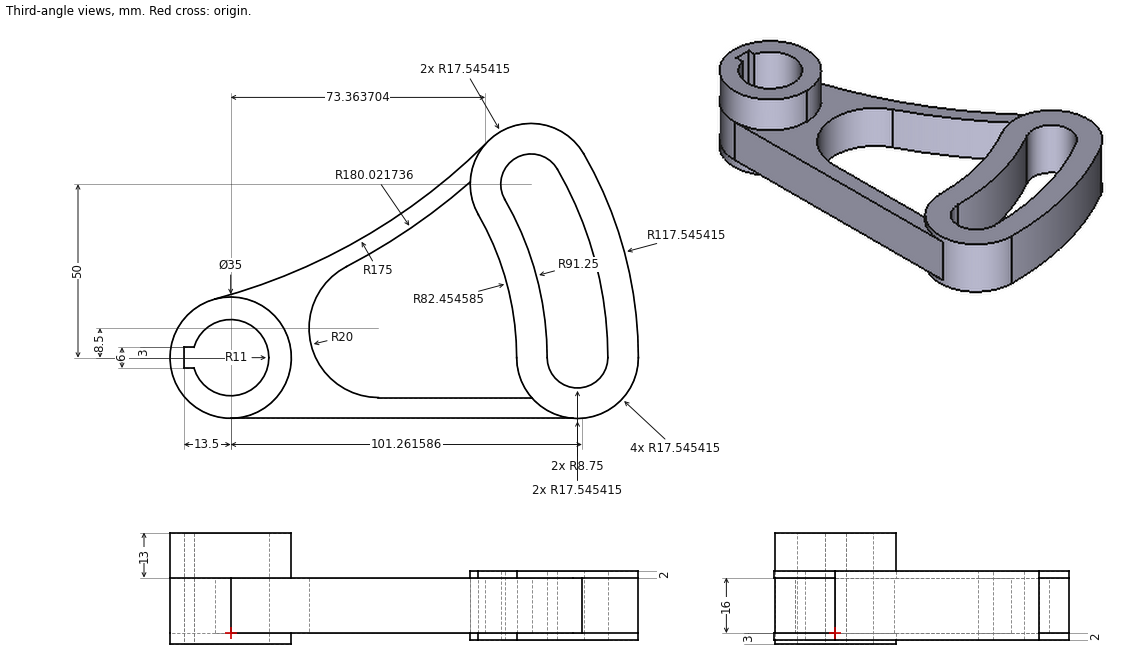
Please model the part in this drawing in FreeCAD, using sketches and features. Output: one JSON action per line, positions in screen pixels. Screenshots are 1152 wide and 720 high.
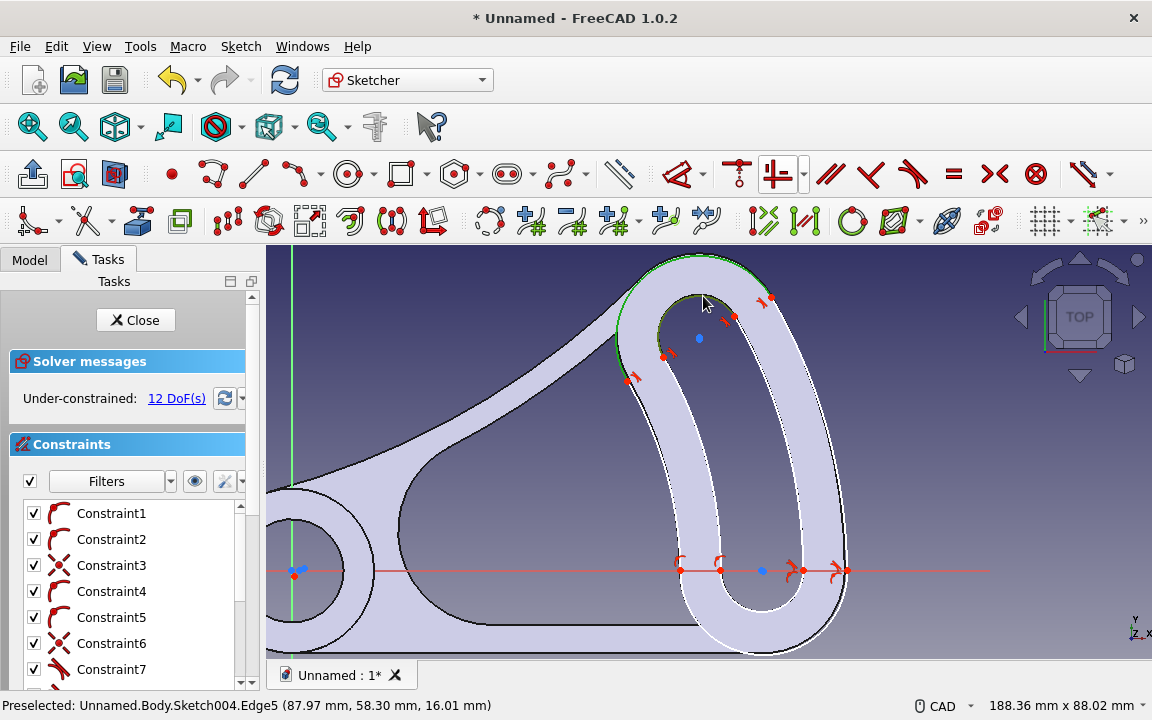
{"action": "left_click", "coordinate": [737, 174]}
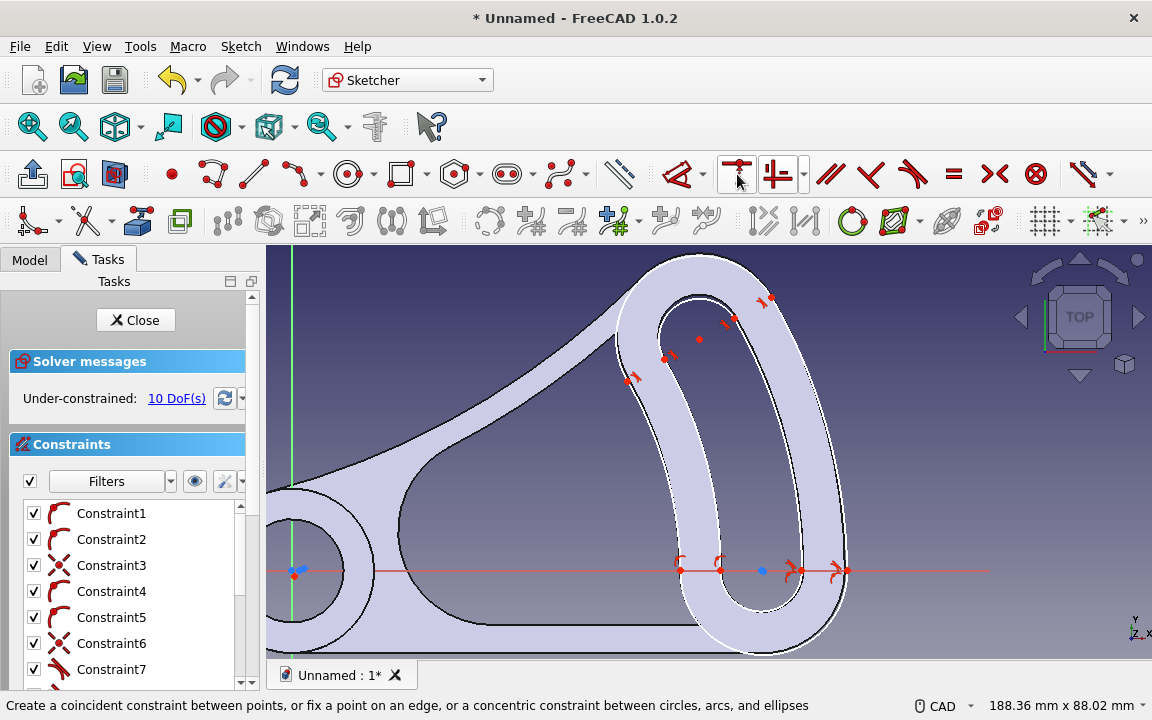
{"action": "left_click", "coordinate": [840, 485]}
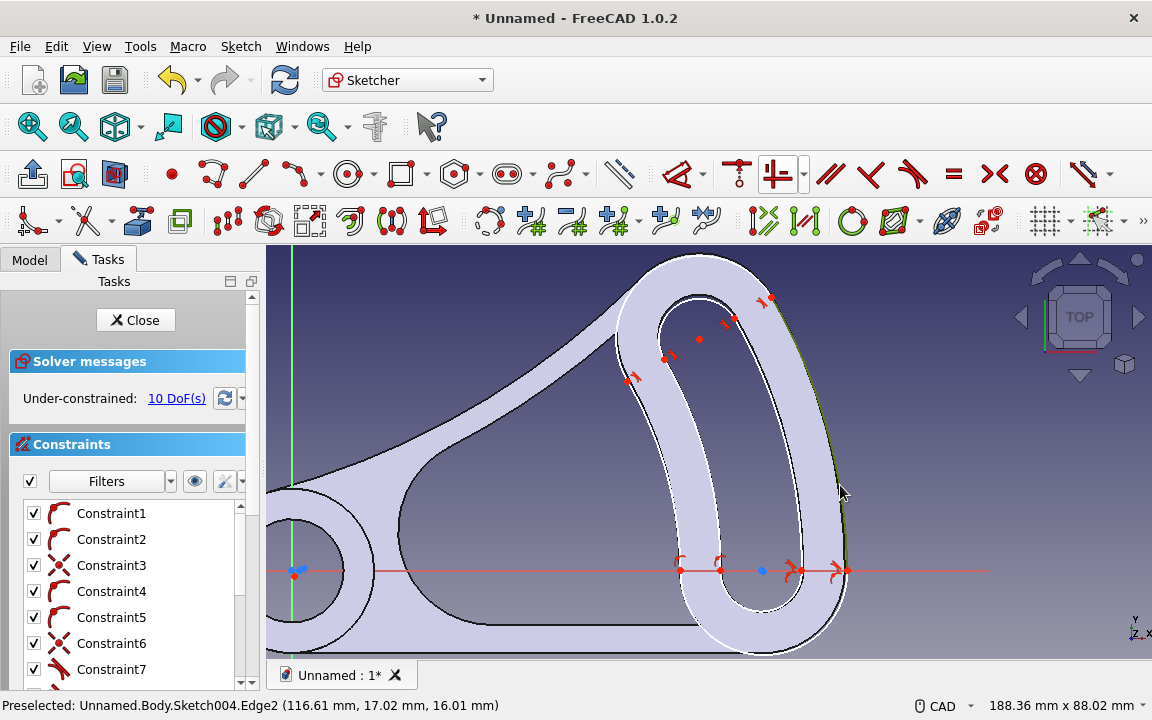
{"action": "left_click", "coordinate": [796, 492]}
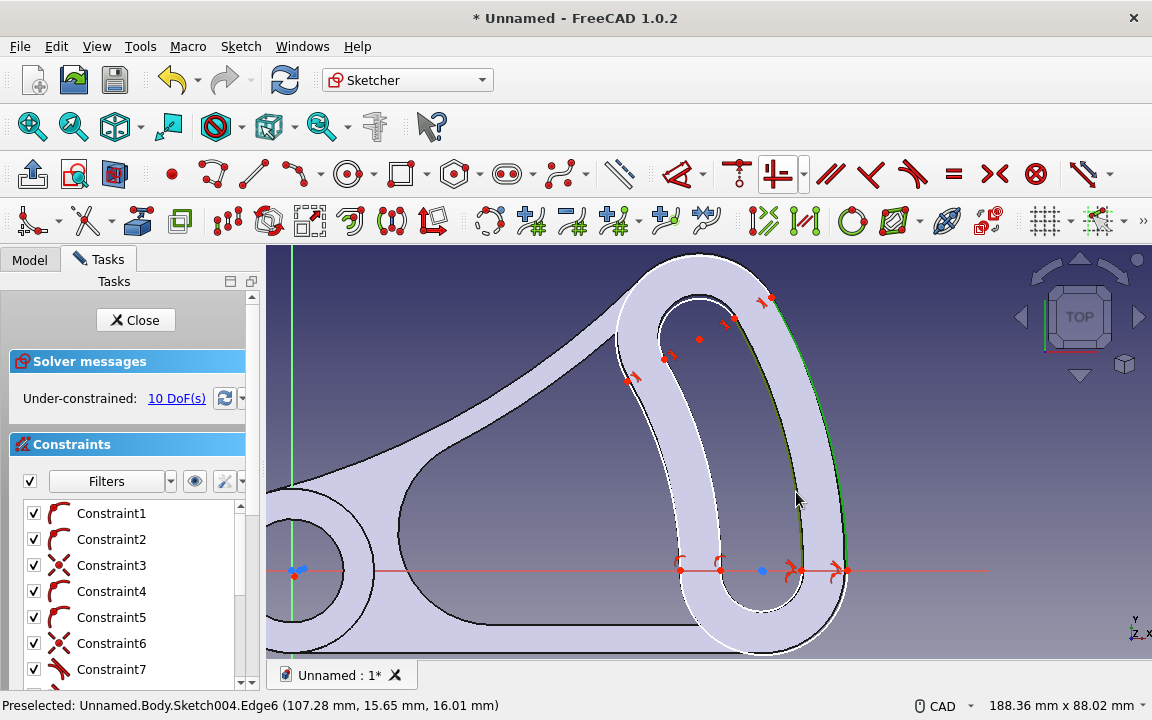
{"action": "left_click", "coordinate": [737, 174]}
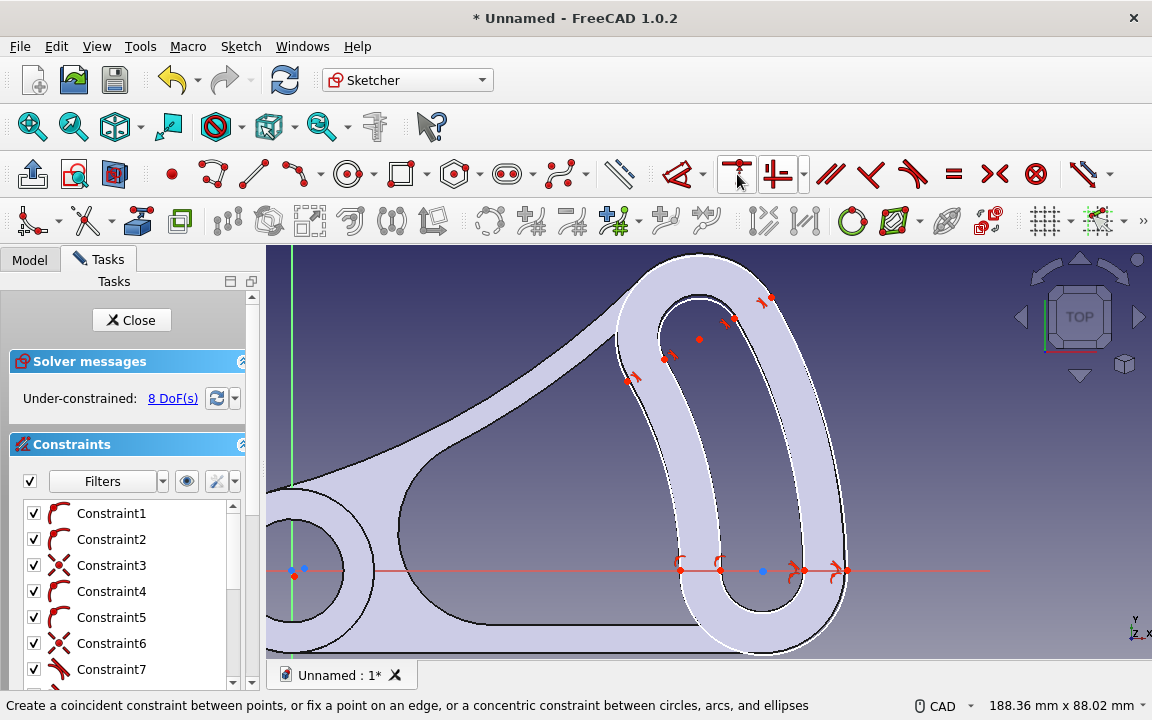
{"action": "left_click", "coordinate": [840, 485]}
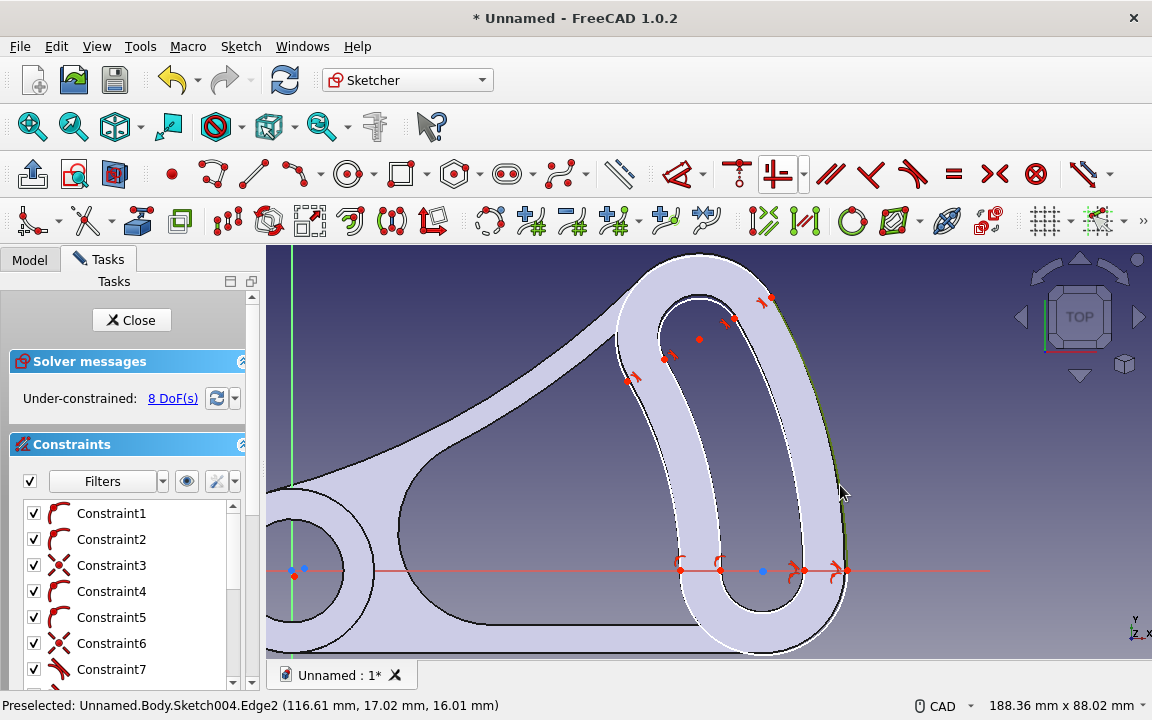
{"action": "left_click", "coordinate": [716, 505]}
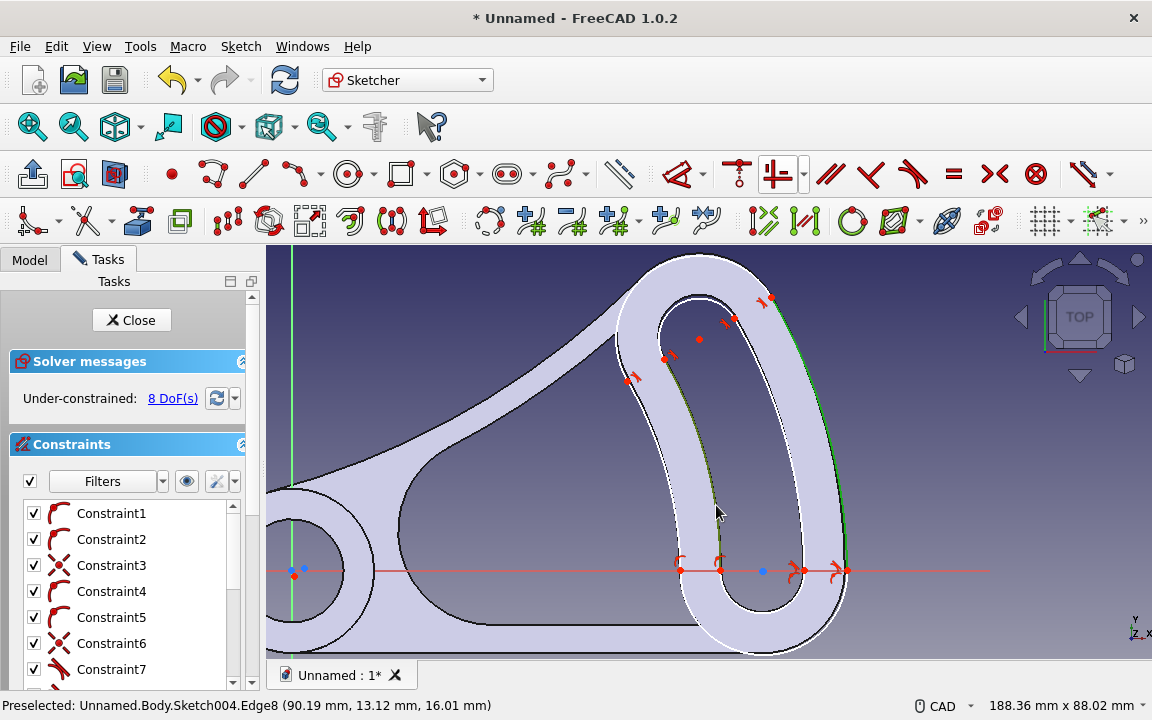
{"action": "left_click", "coordinate": [737, 174]}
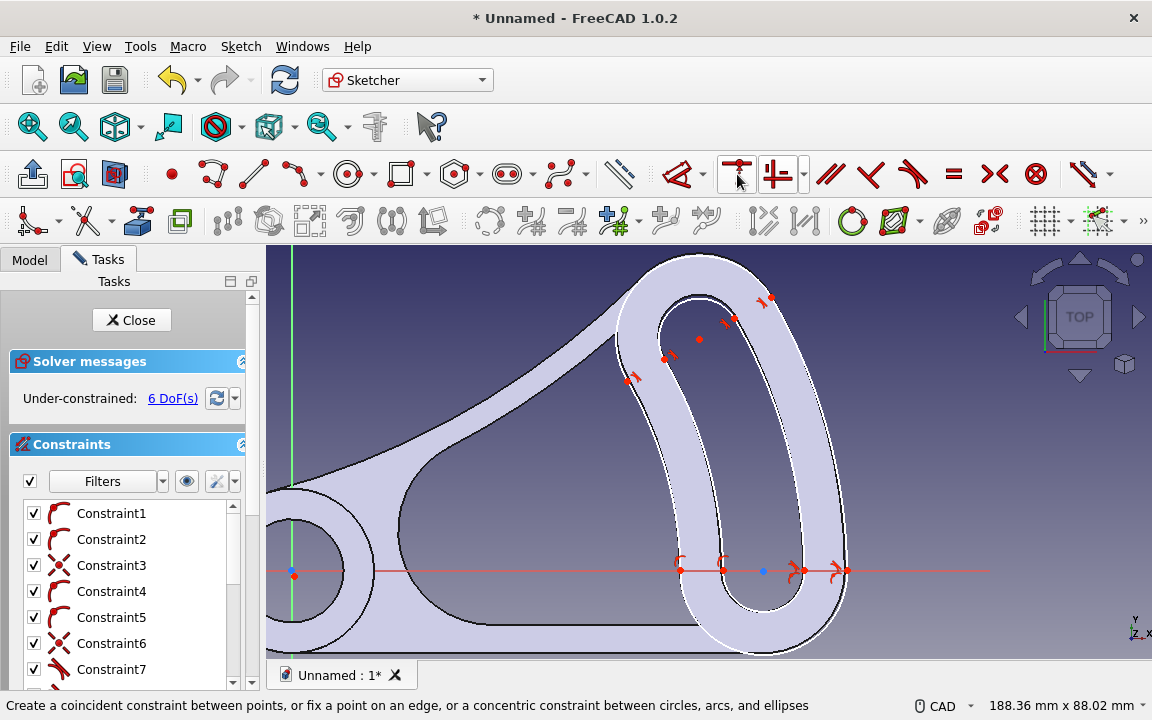
{"action": "scroll", "coordinate": [787, 438], "scroll_direction": "down", "scroll_amount": 2}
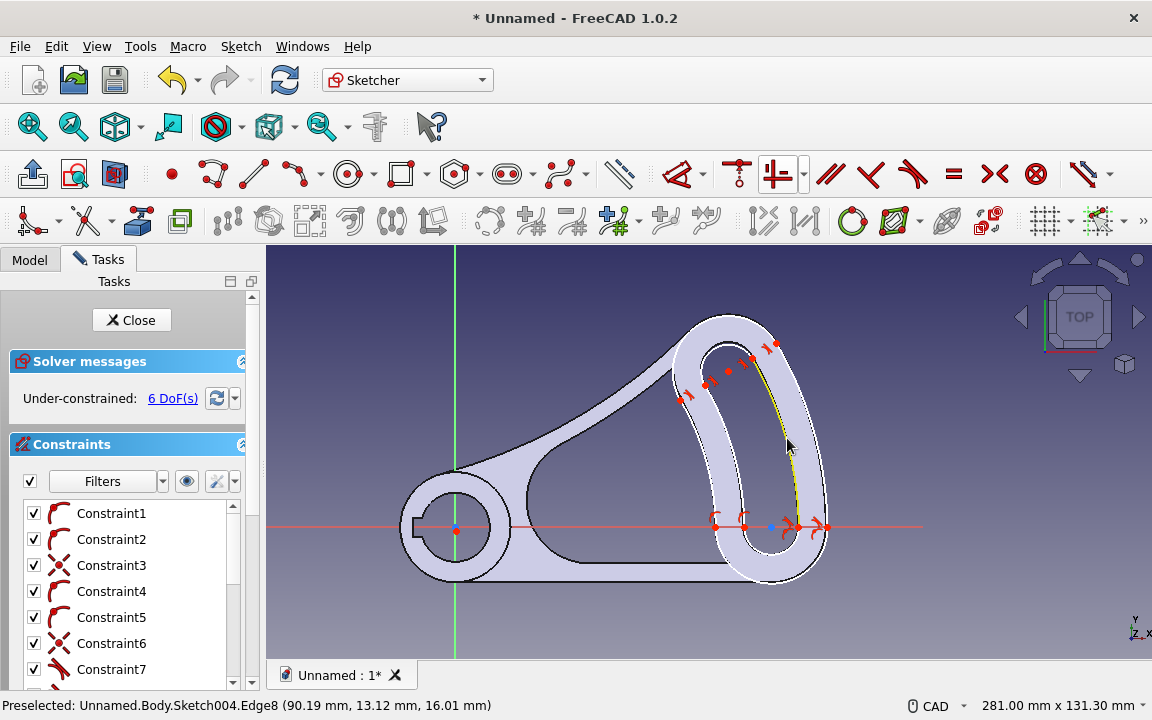
{"action": "scroll", "coordinate": [456, 529], "scroll_direction": "up", "scroll_amount": 2}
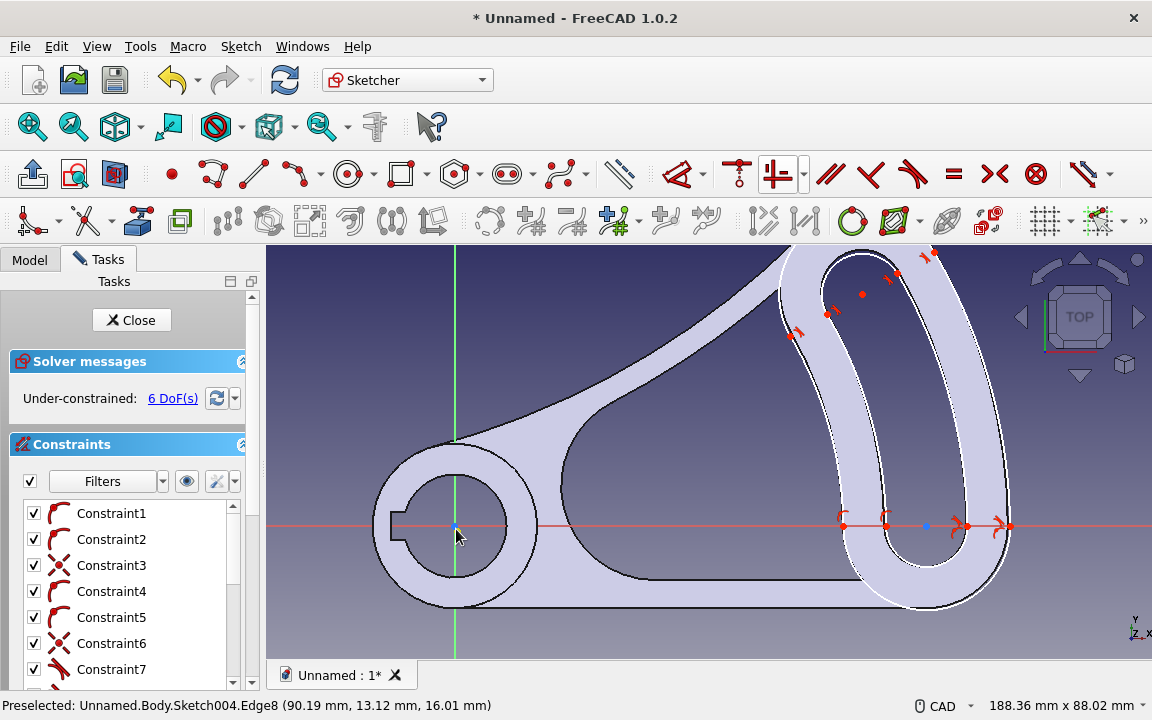
{"action": "left_click_drag", "start_coordinate": [445, 516], "coordinate": [467, 542]}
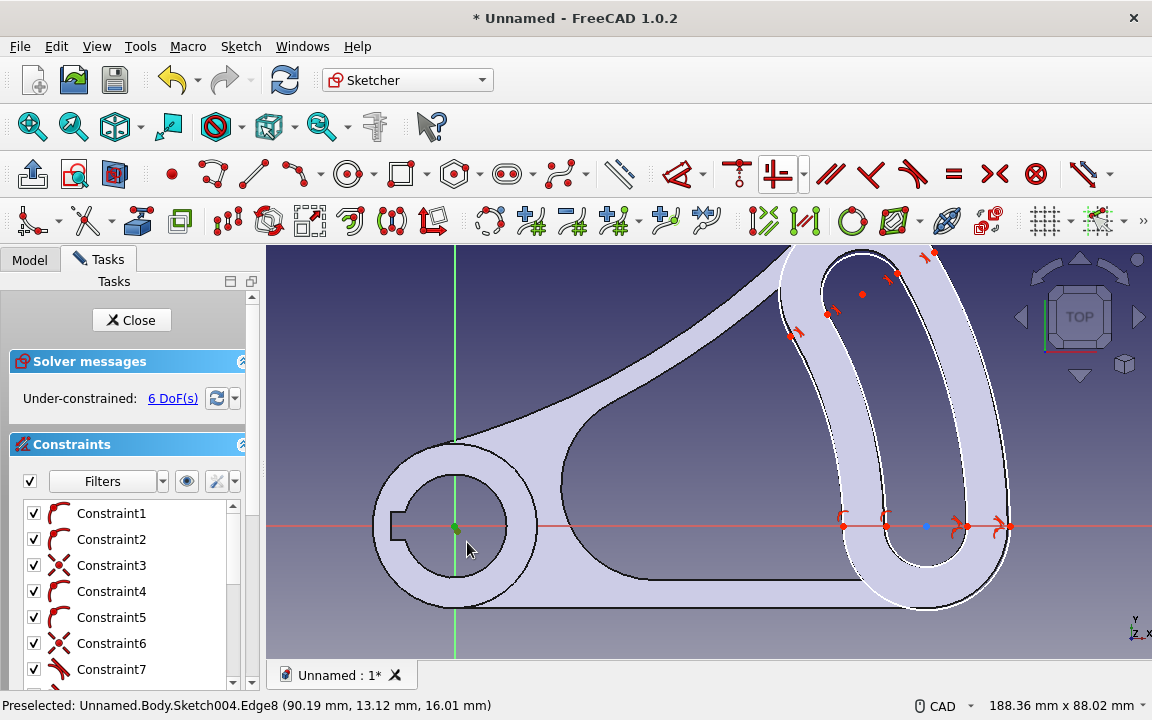
{"action": "left_click", "coordinate": [737, 174]}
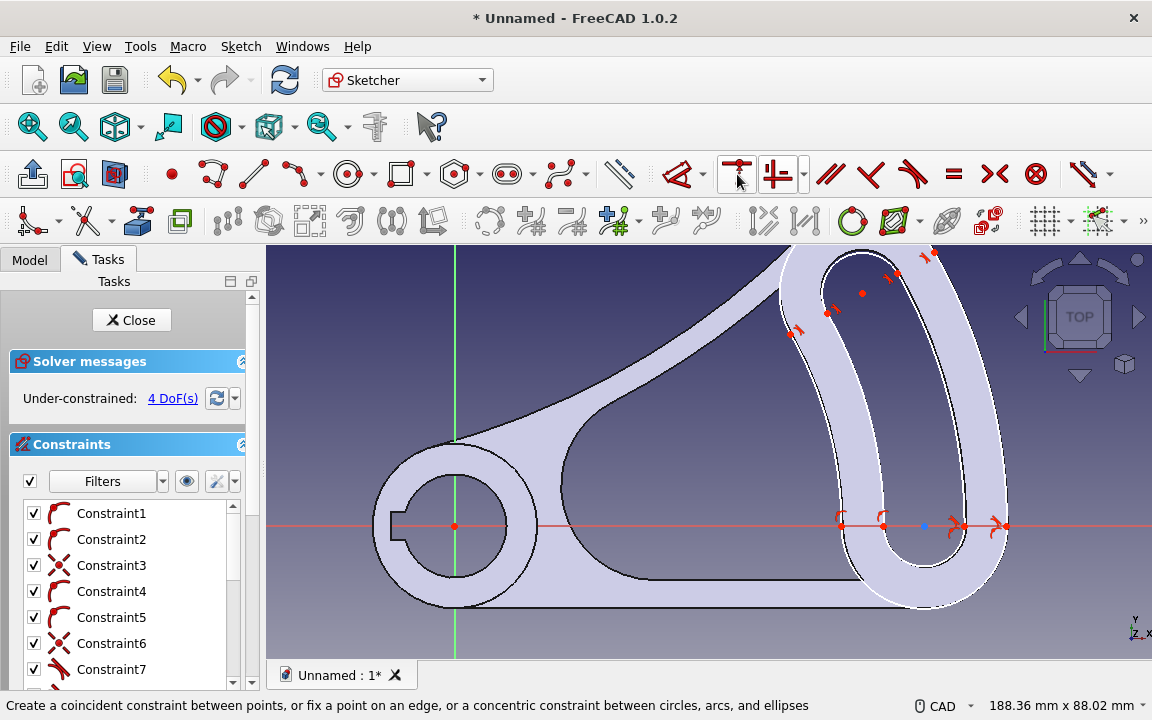
{"action": "left_click", "coordinate": [676, 174]}